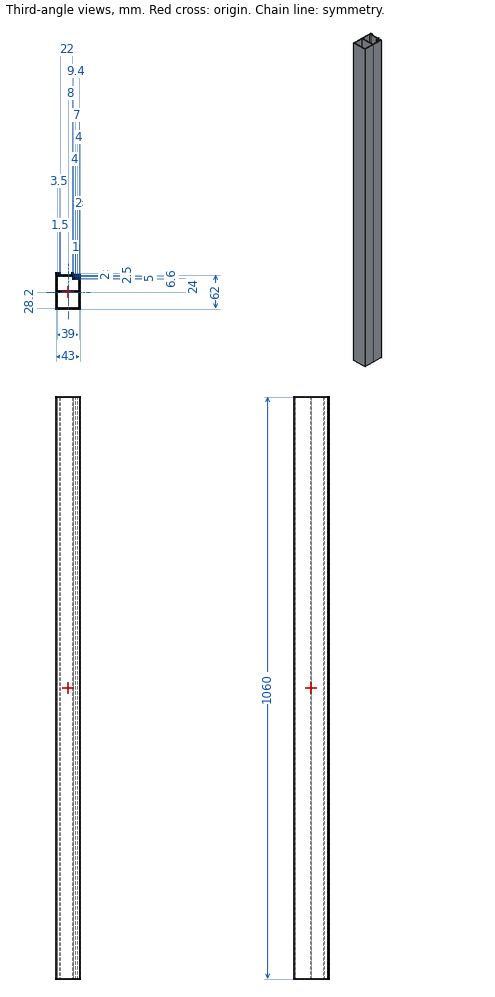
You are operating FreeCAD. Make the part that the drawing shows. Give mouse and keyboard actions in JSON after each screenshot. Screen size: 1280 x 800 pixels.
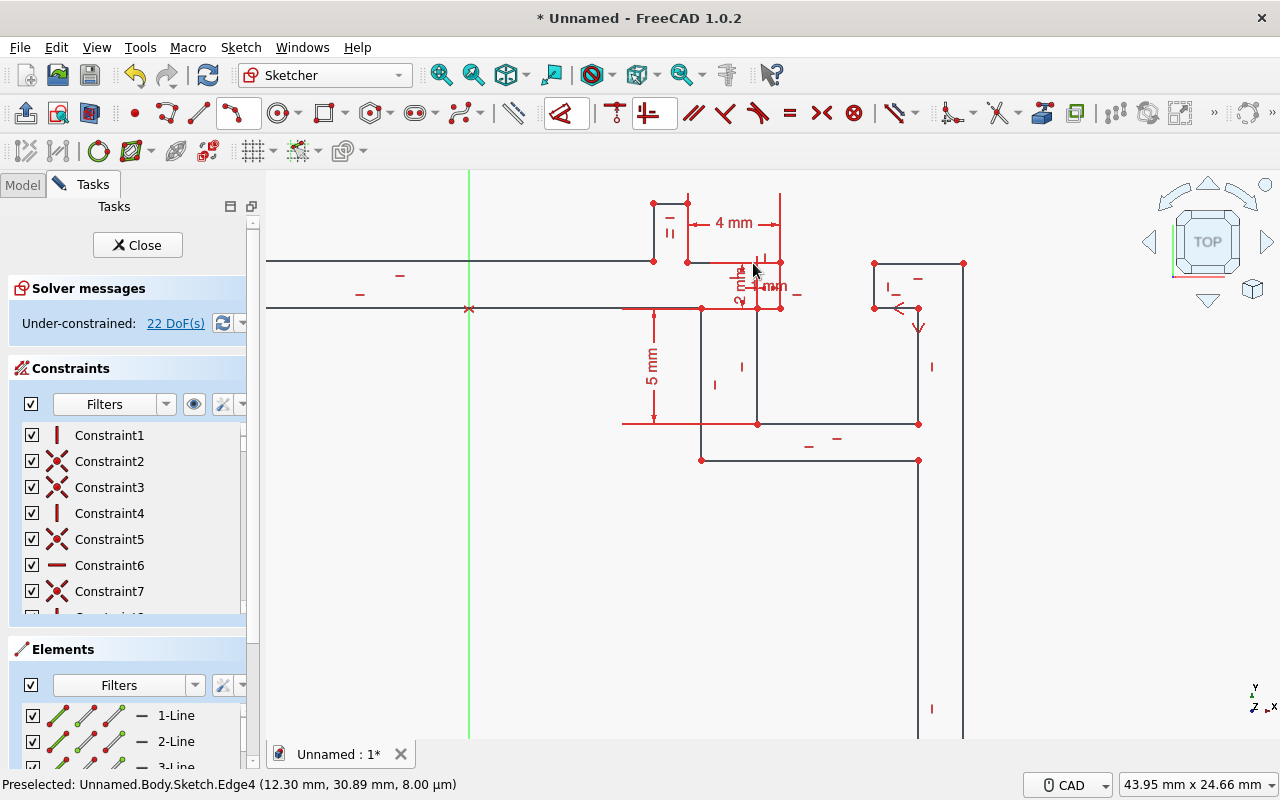
{"action": "left_click", "coordinate": [937, 264]}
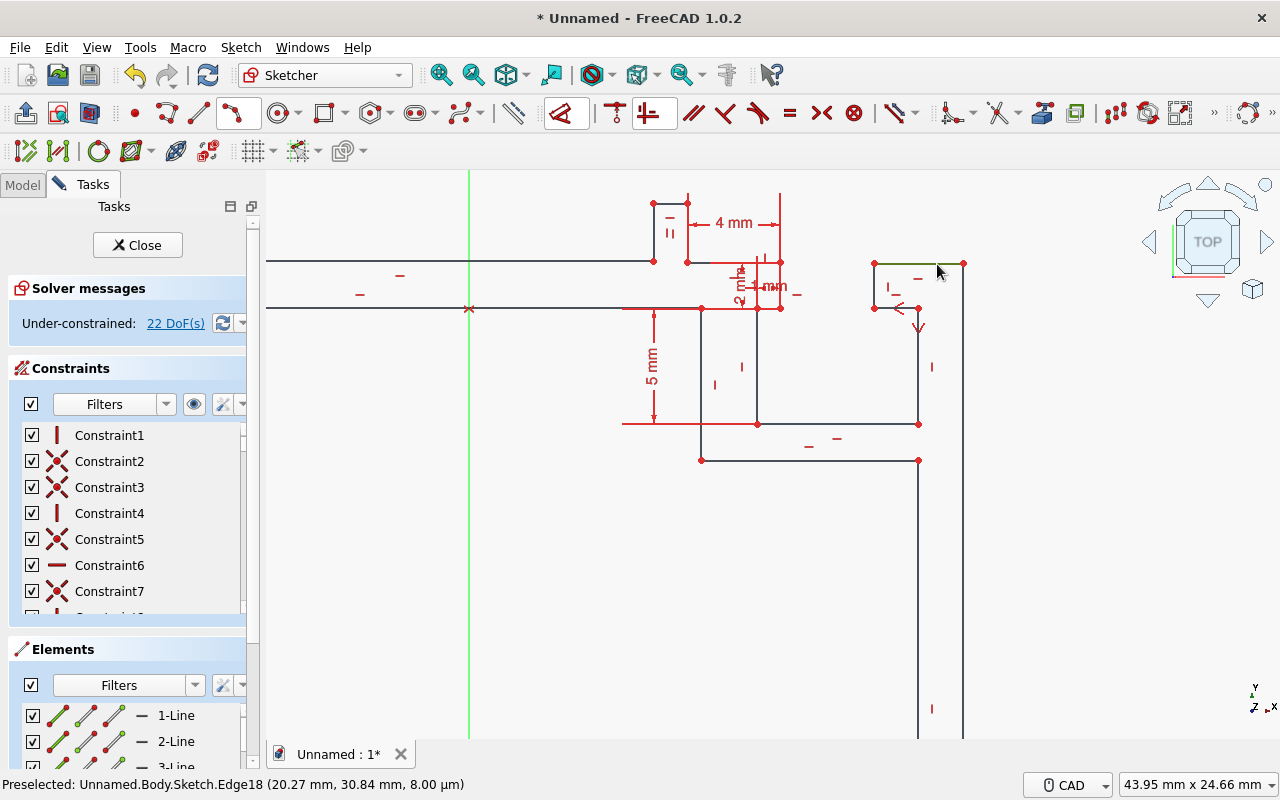
{"action": "left_click", "coordinate": [584, 114]}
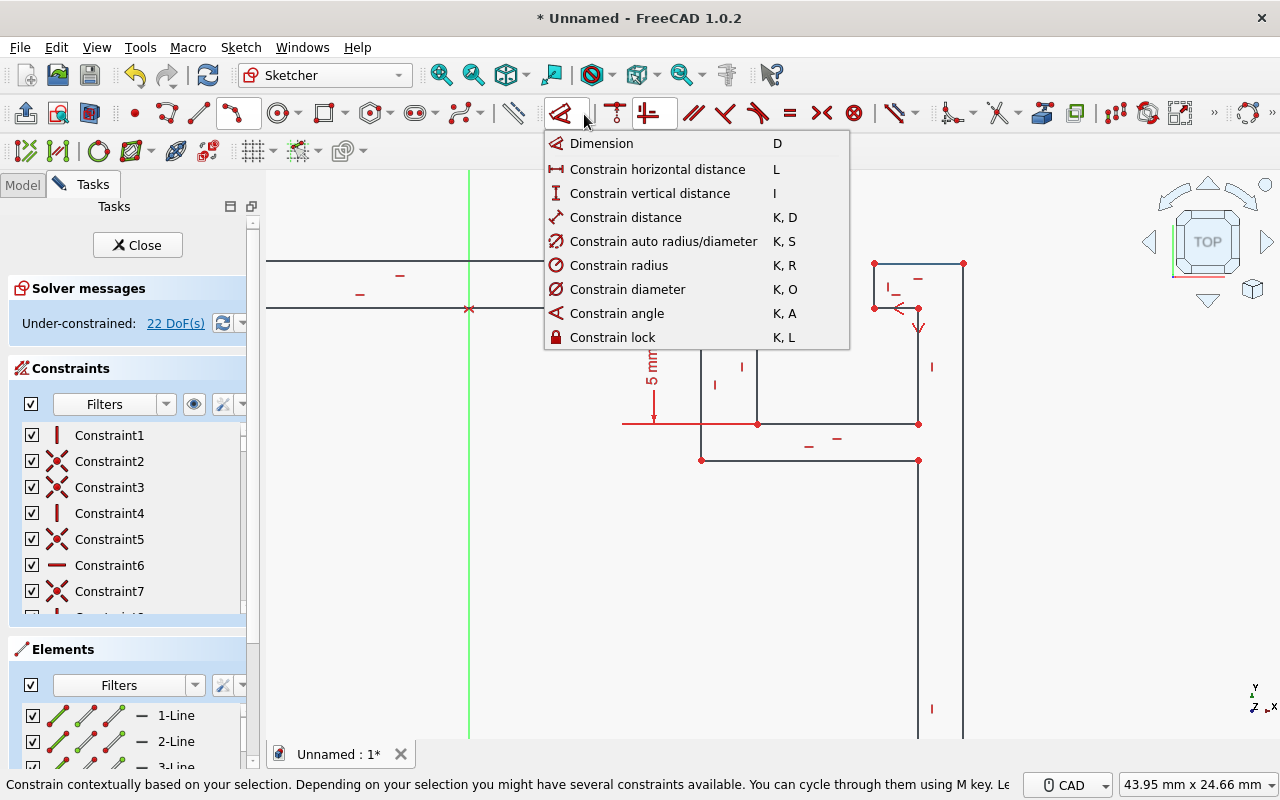
{"action": "left_click", "coordinate": [697, 169]}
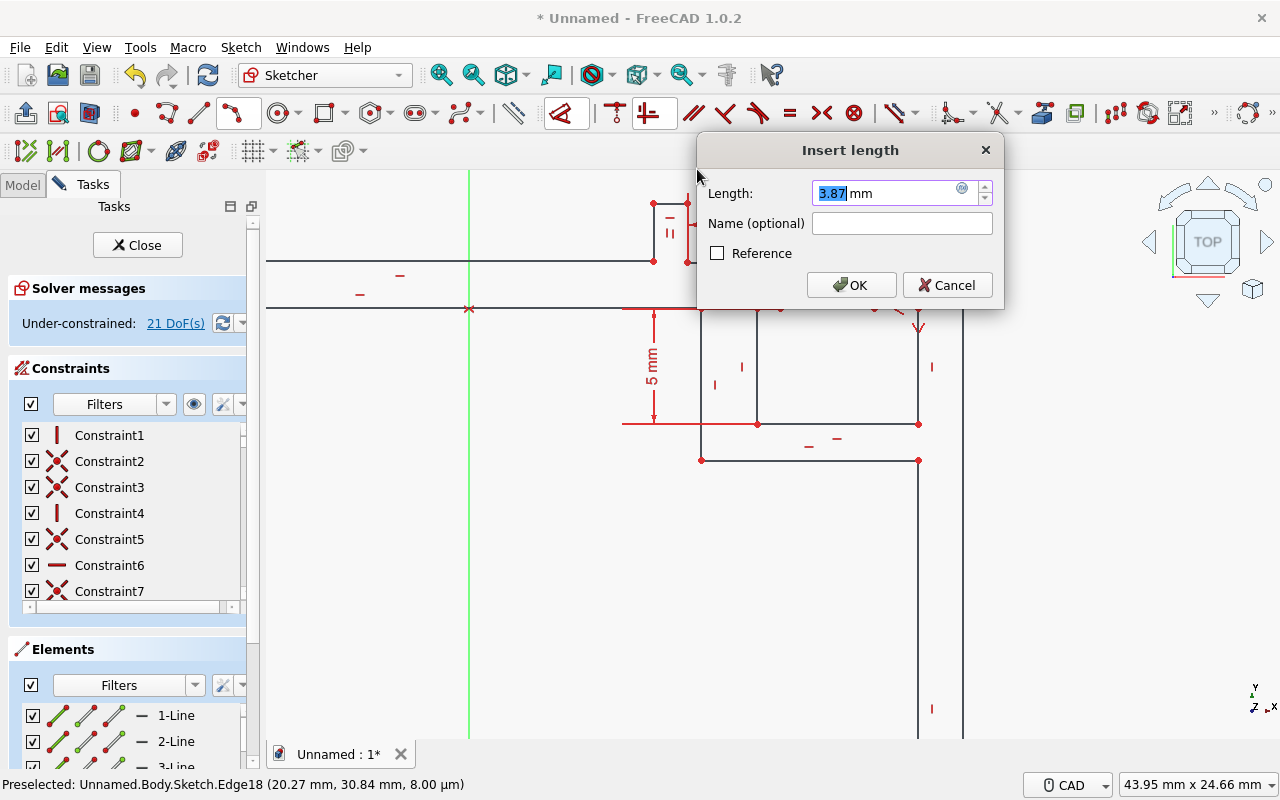
{"action": "type", "text": "4"}
{"action": "key", "text": "Return"}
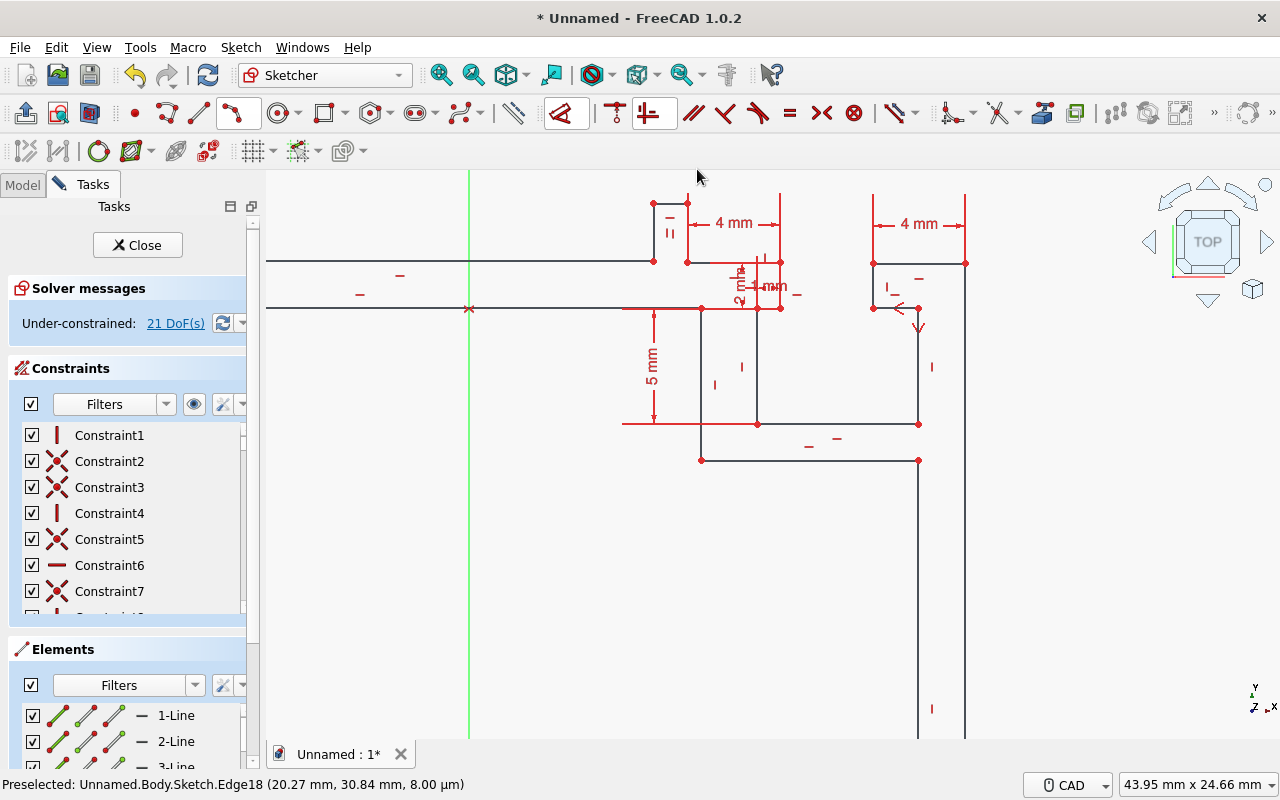
{"action": "left_click", "coordinate": [873, 277]}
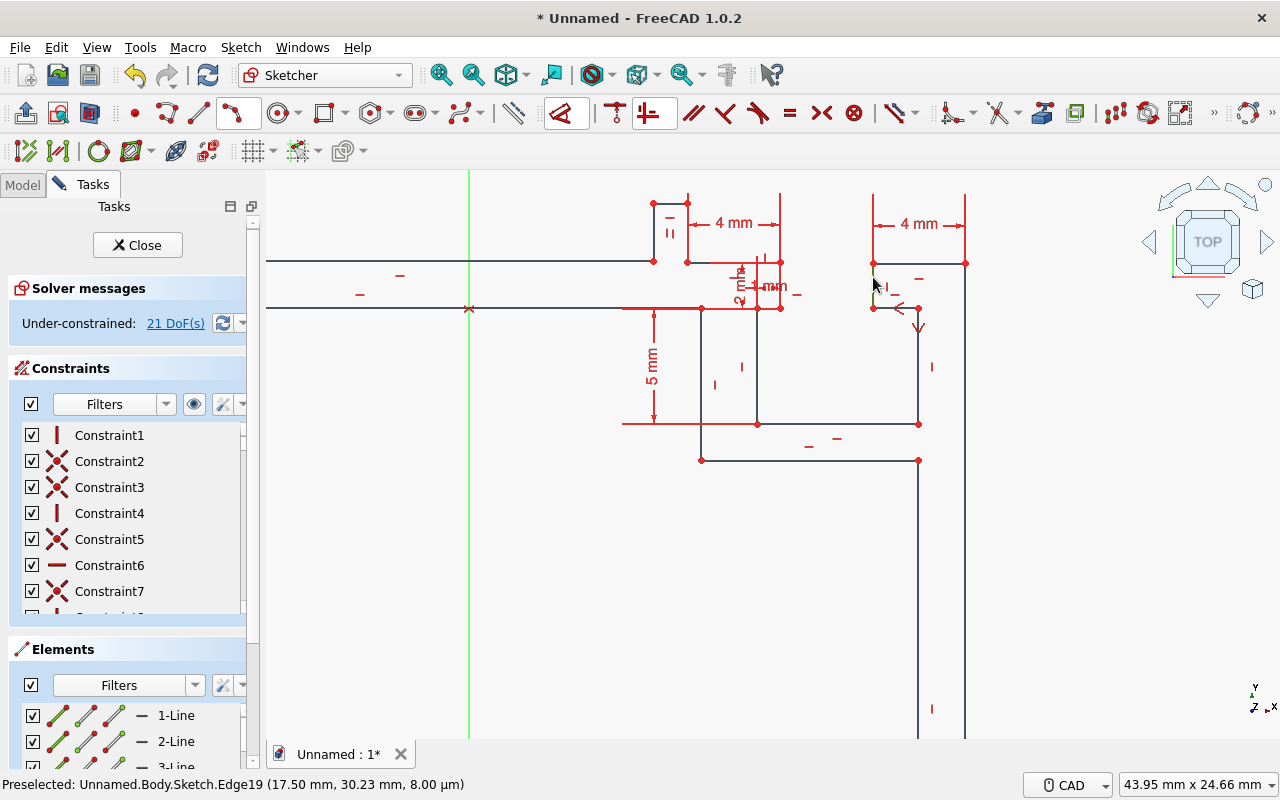
{"action": "key", "text": "i"}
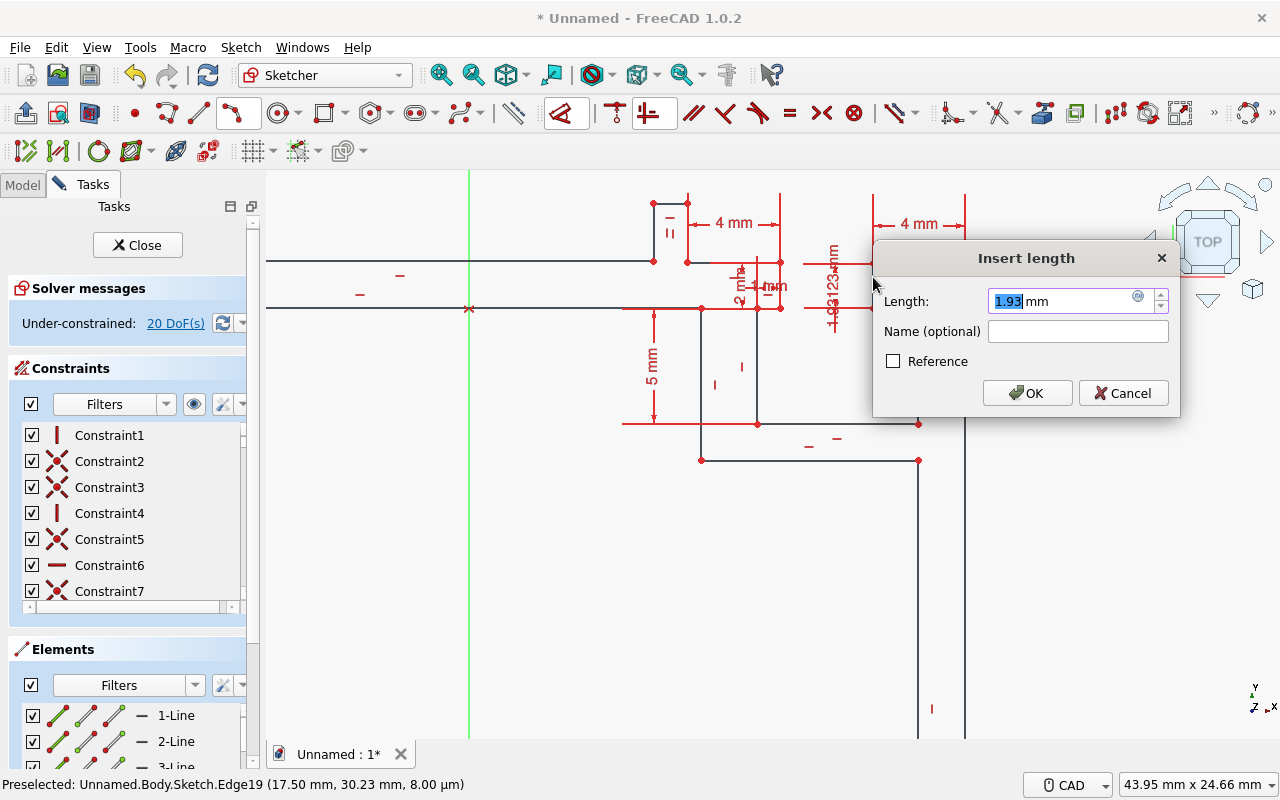
{"action": "type", "text": "2"}
{"action": "key", "text": "Return"}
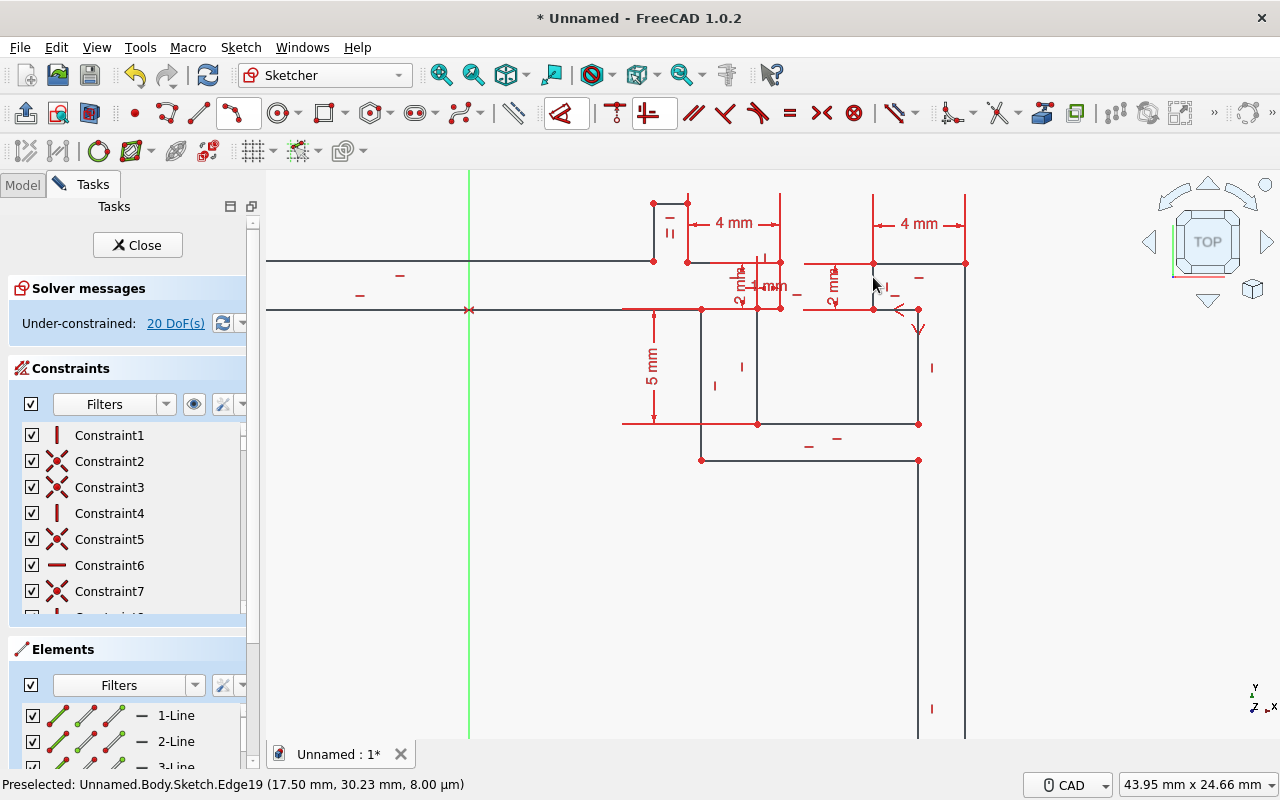
{"action": "left_click", "coordinate": [887, 310]}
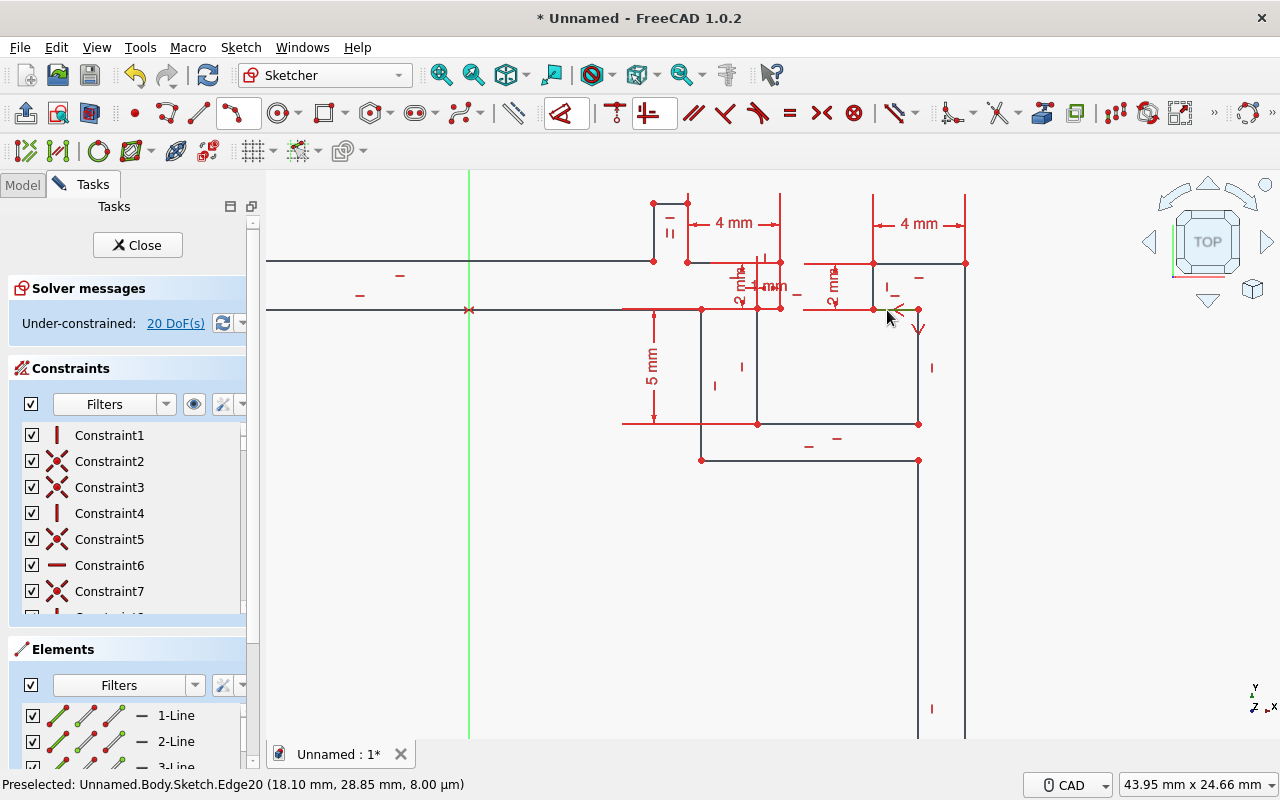
{"action": "key", "text": "l"}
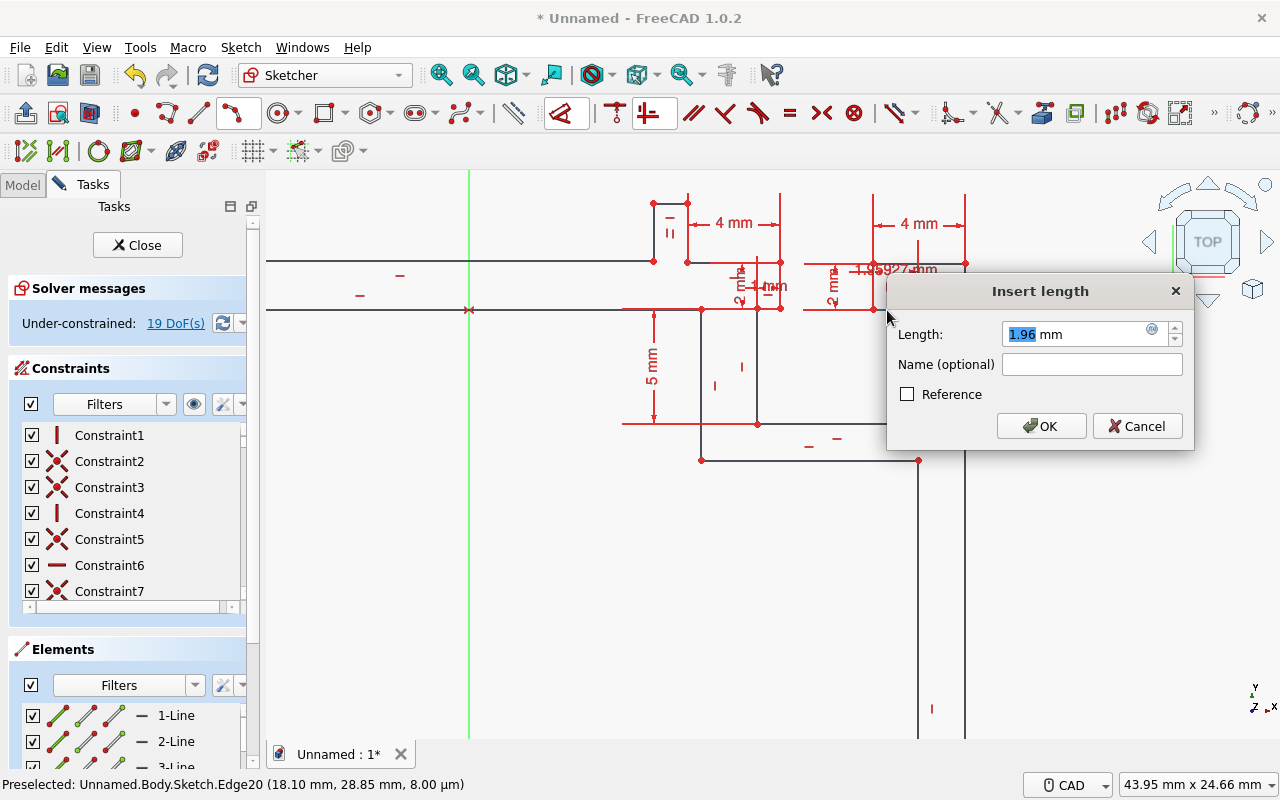
{"action": "type", "text": "2"}
{"action": "key", "text": "Return"}